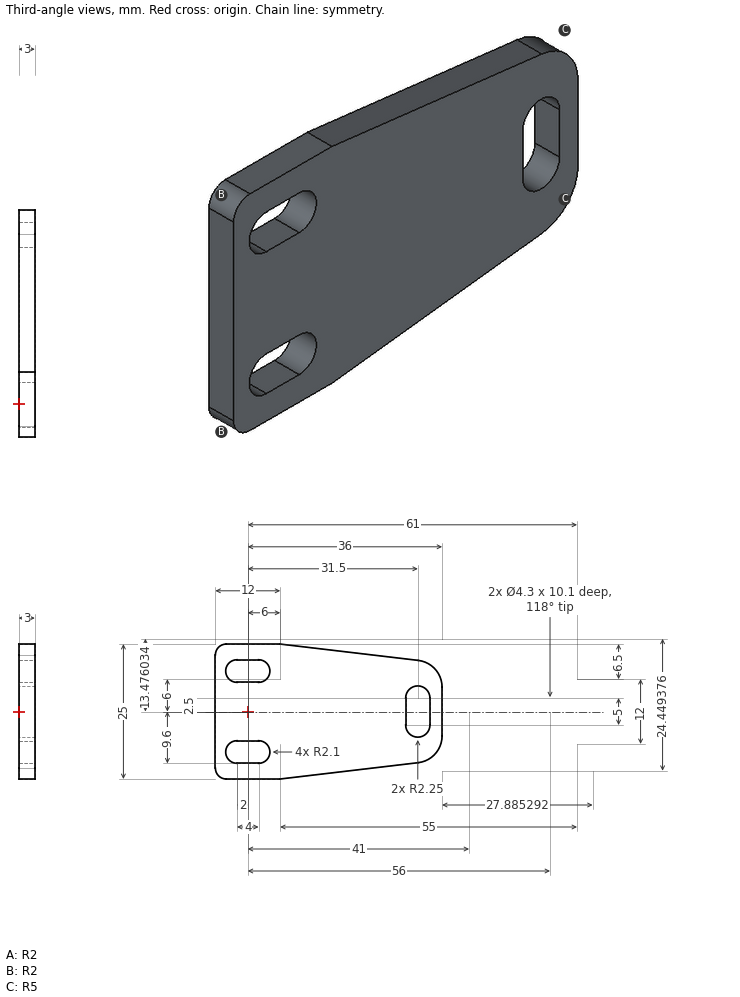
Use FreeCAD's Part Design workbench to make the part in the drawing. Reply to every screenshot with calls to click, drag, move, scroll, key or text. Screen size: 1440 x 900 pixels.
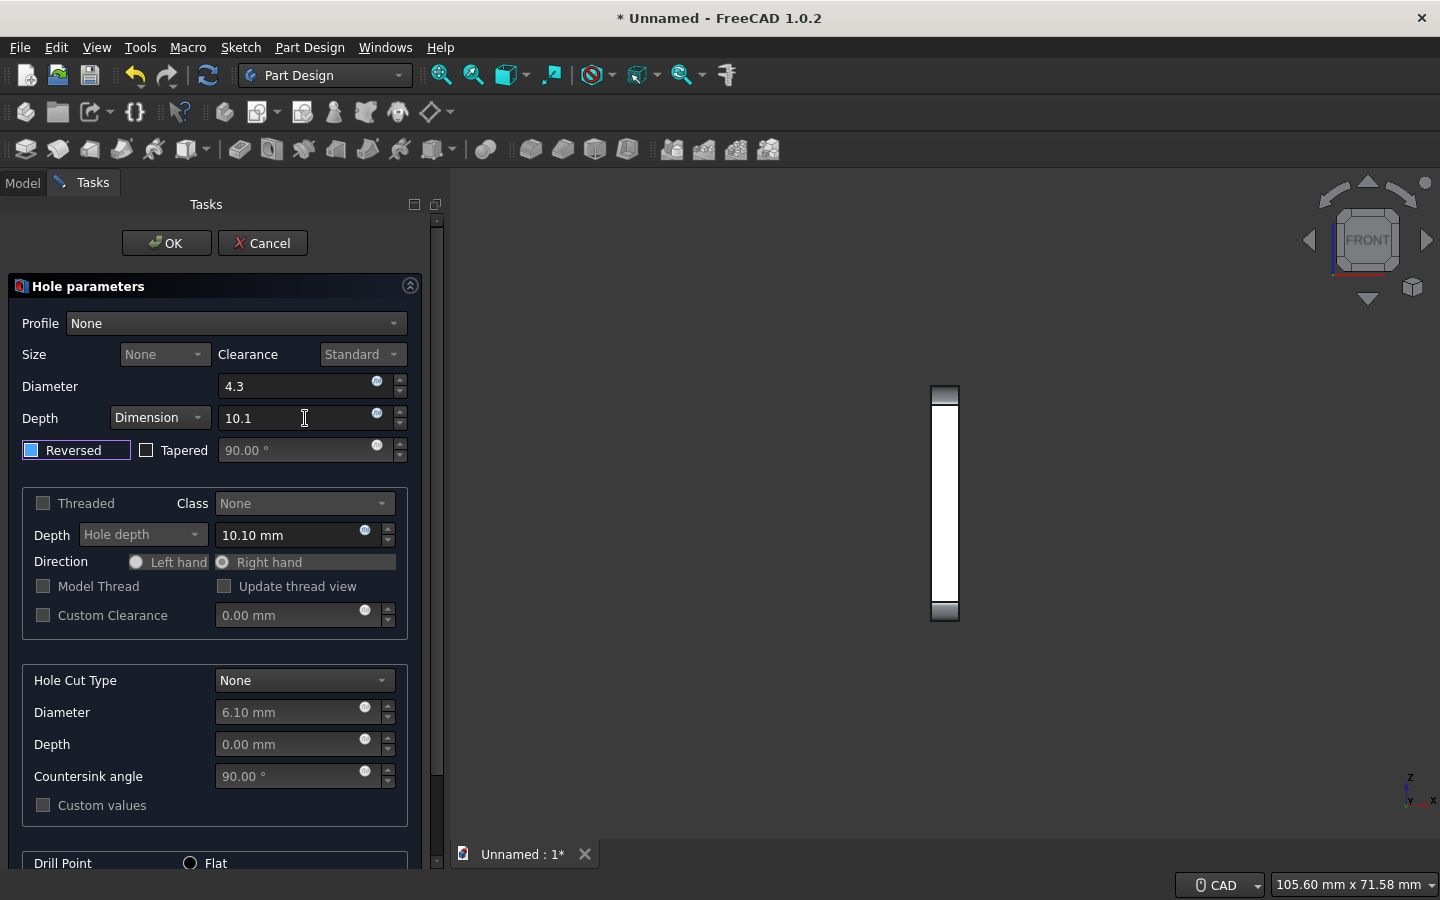
click(30, 450)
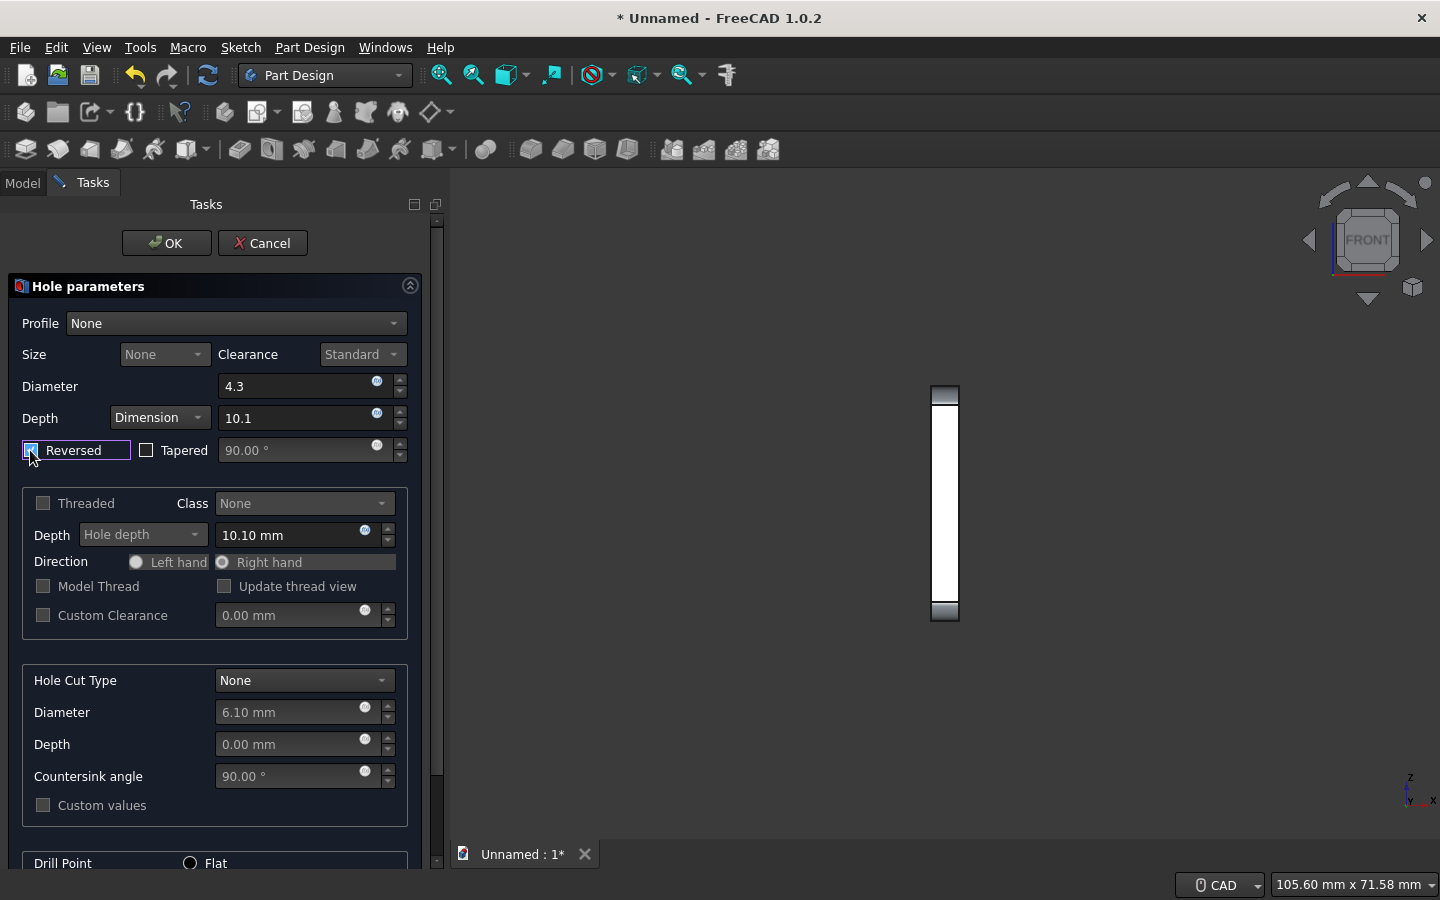
click(167, 243)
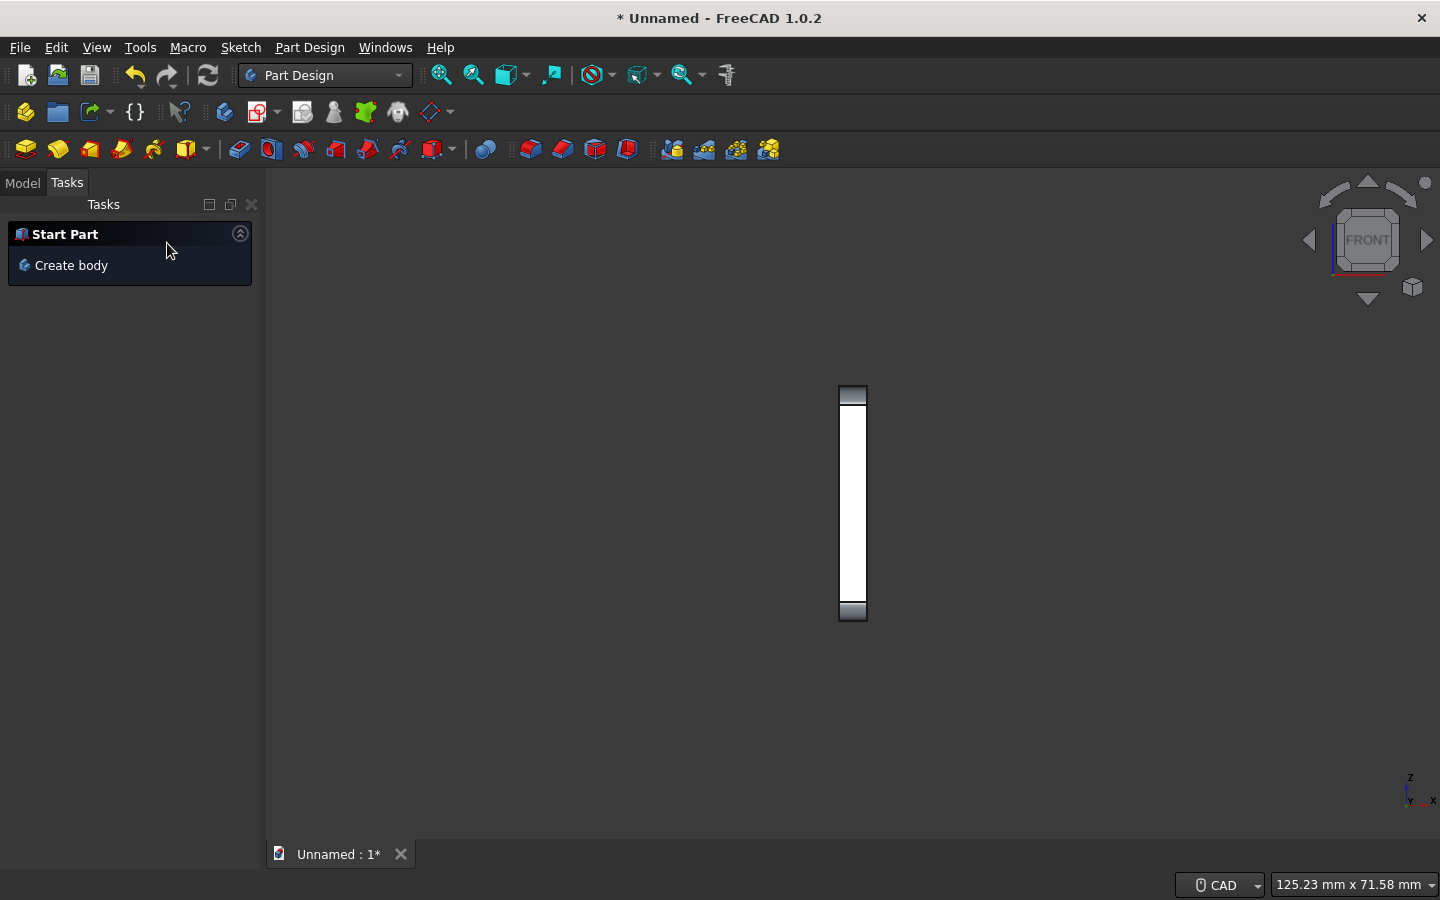
key(v)
key(f)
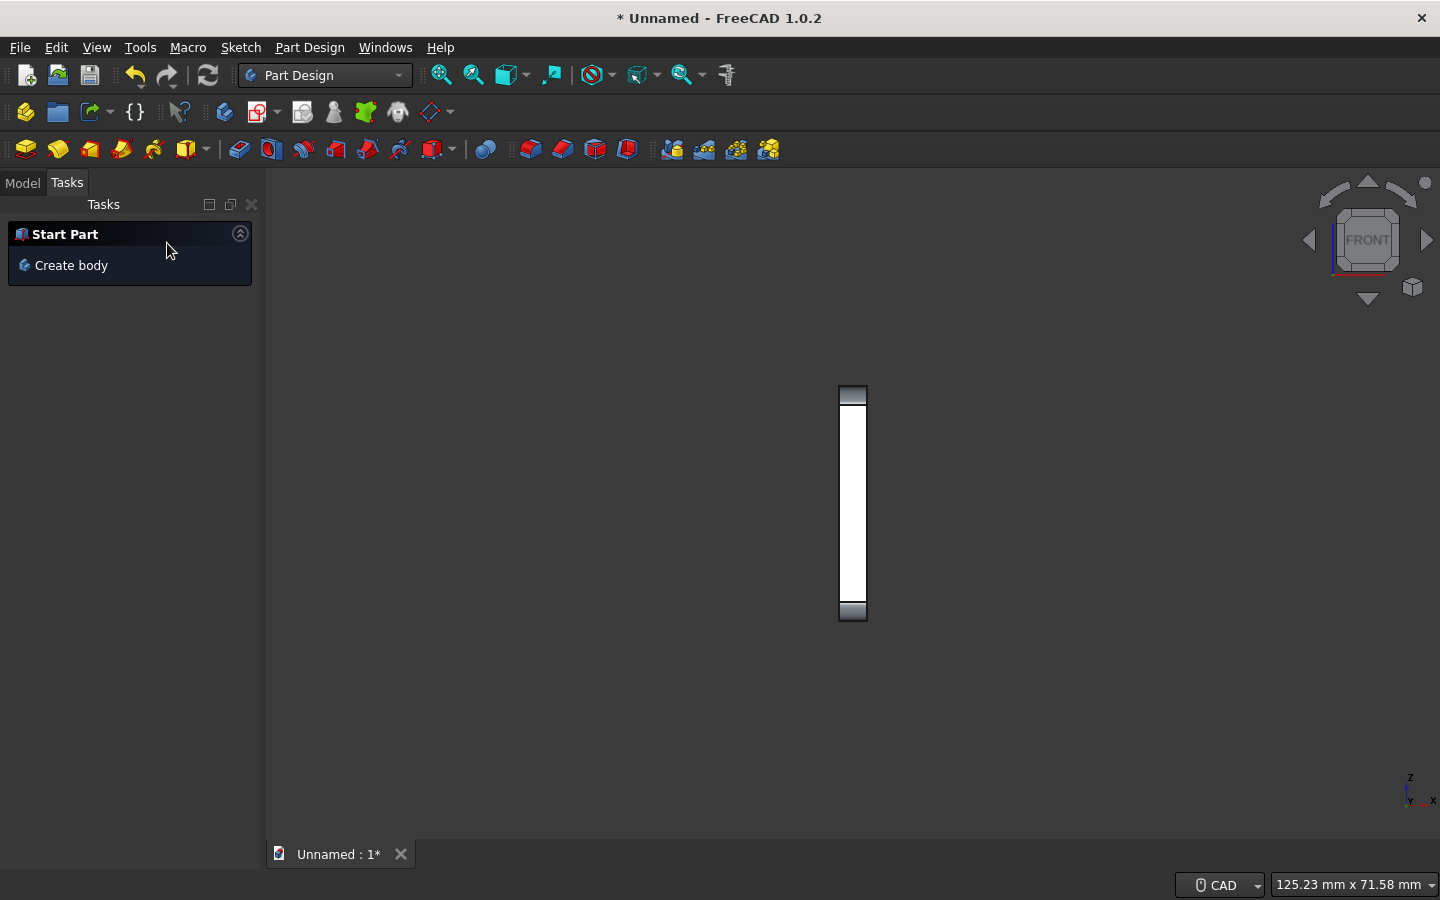
key(0)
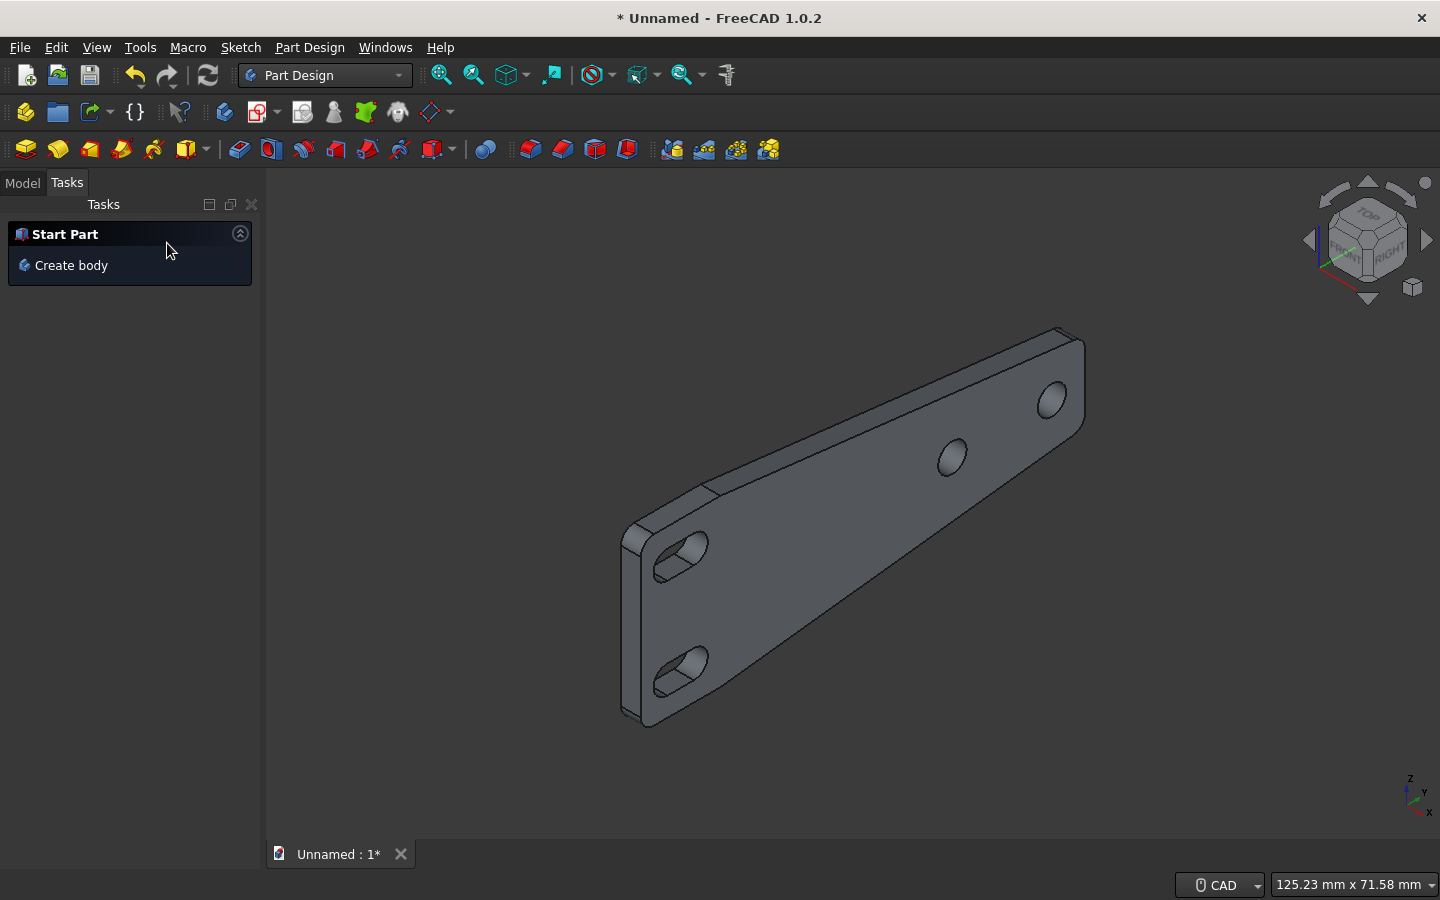
click(799, 545)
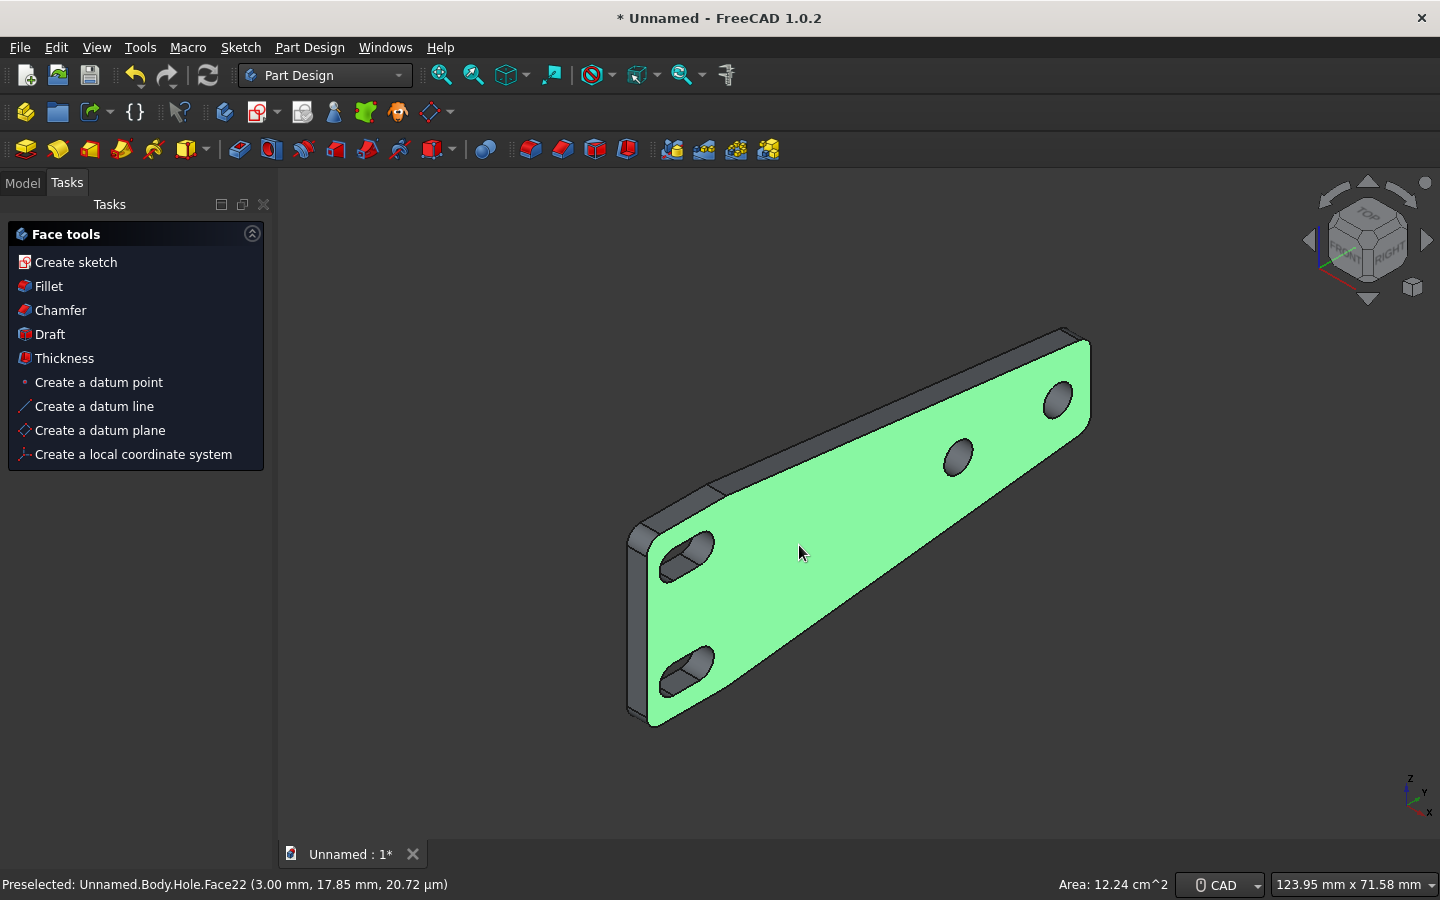
click(258, 112)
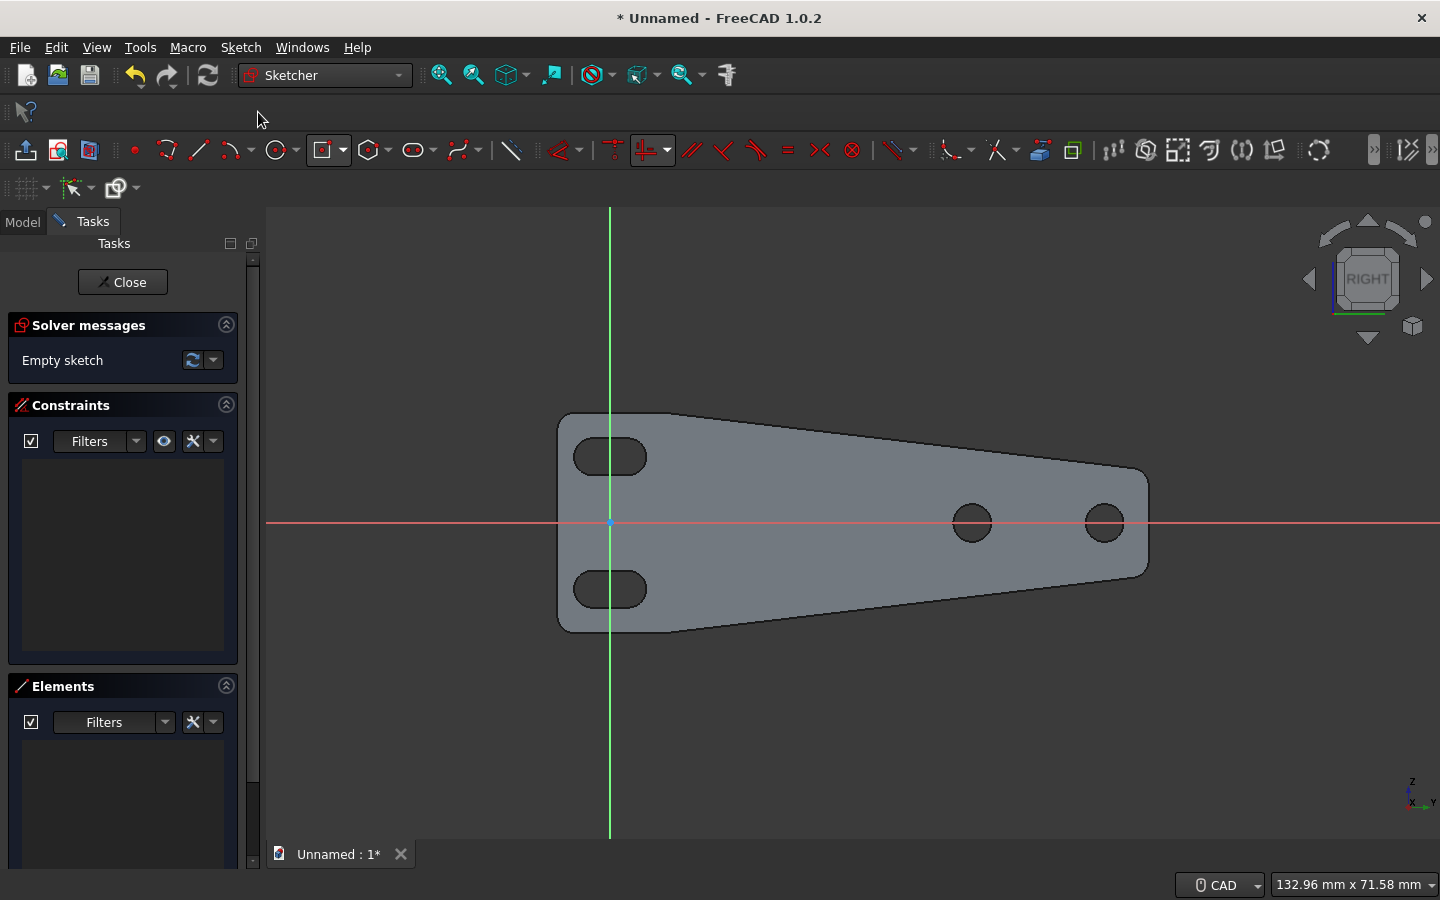
click(346, 150)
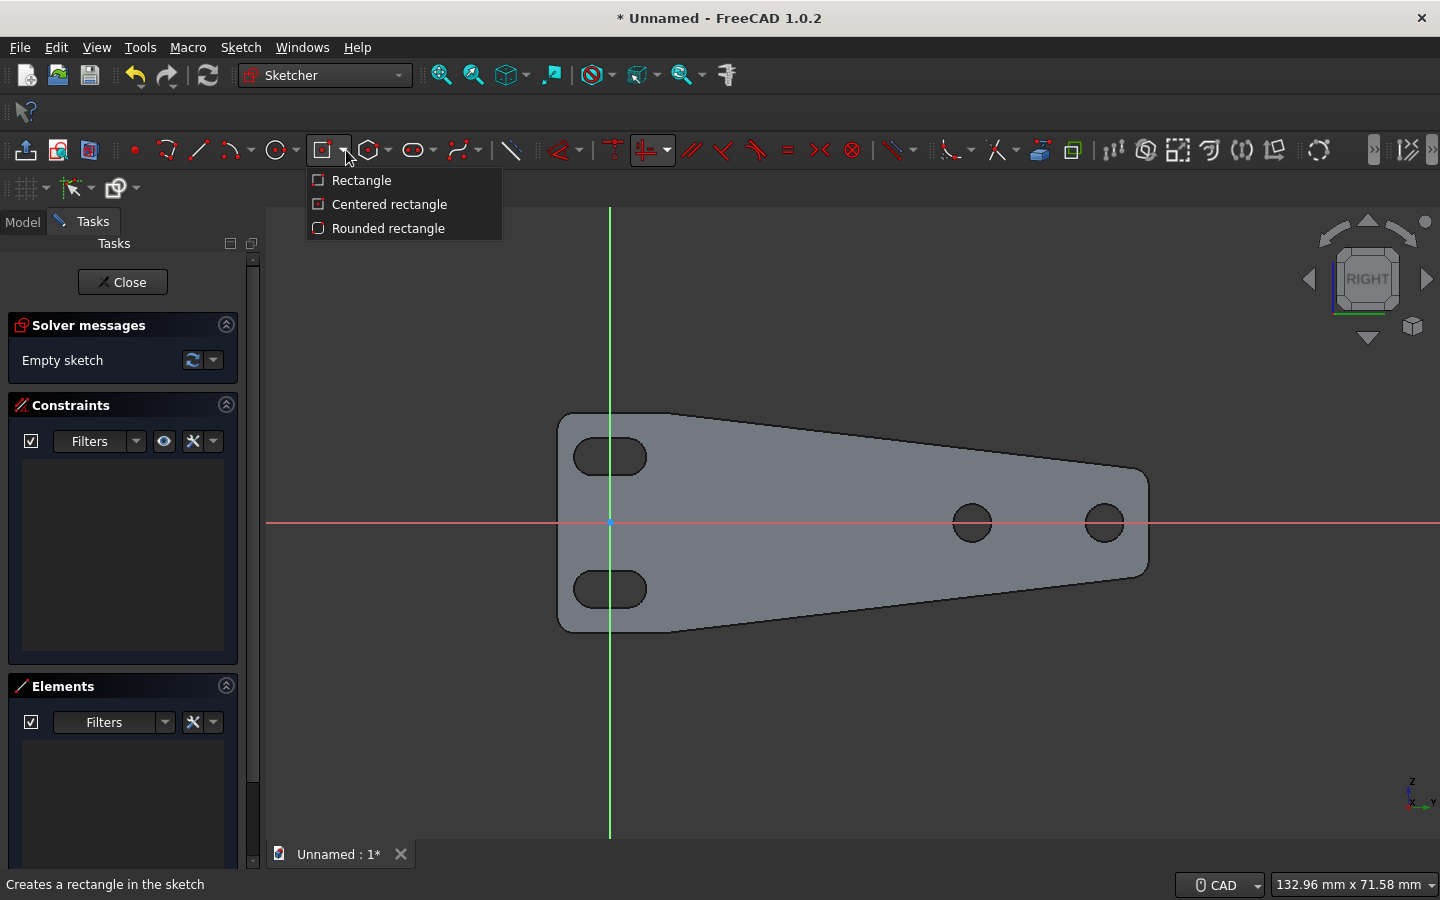
click(404, 180)